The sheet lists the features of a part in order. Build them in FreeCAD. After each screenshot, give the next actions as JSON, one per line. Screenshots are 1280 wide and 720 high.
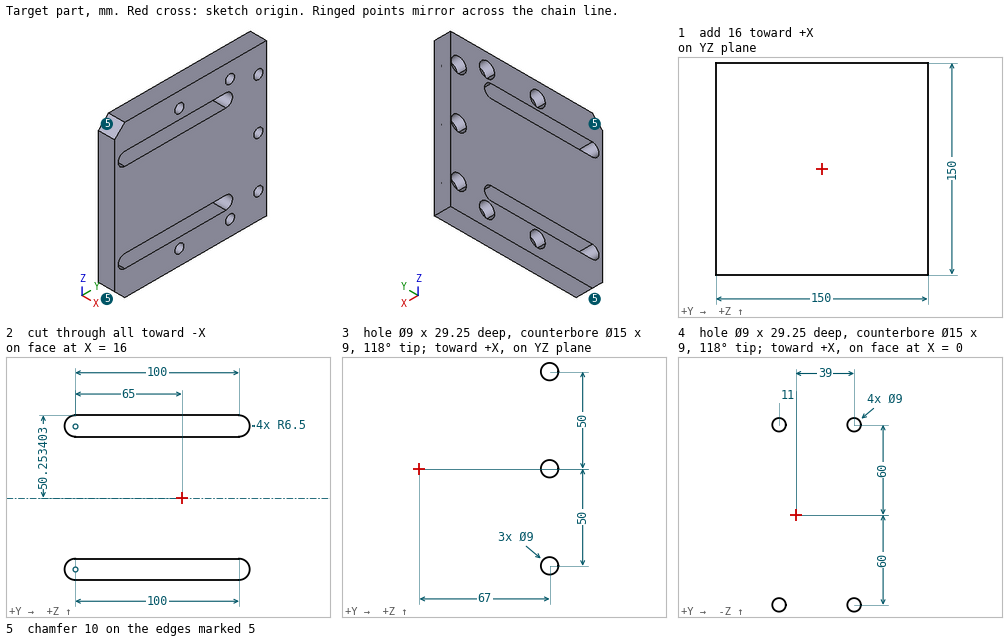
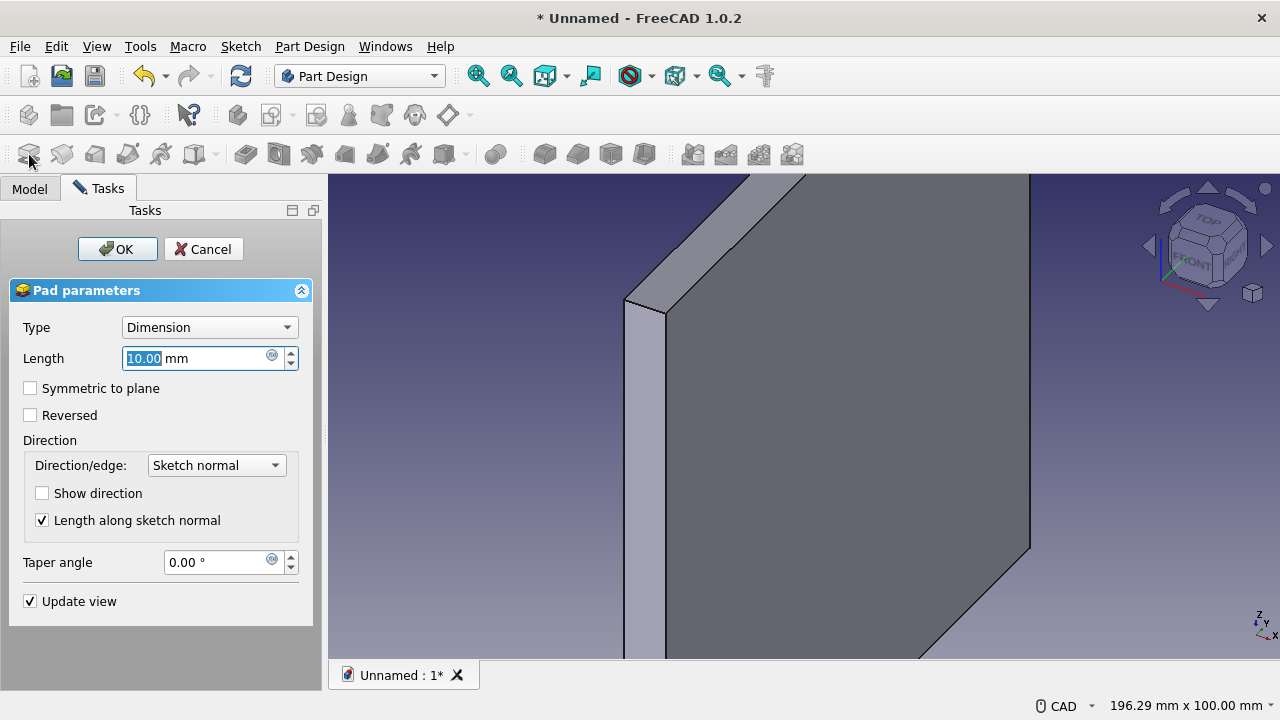
{"action": "type", "text": "16"}
{"action": "key", "text": "Tab"}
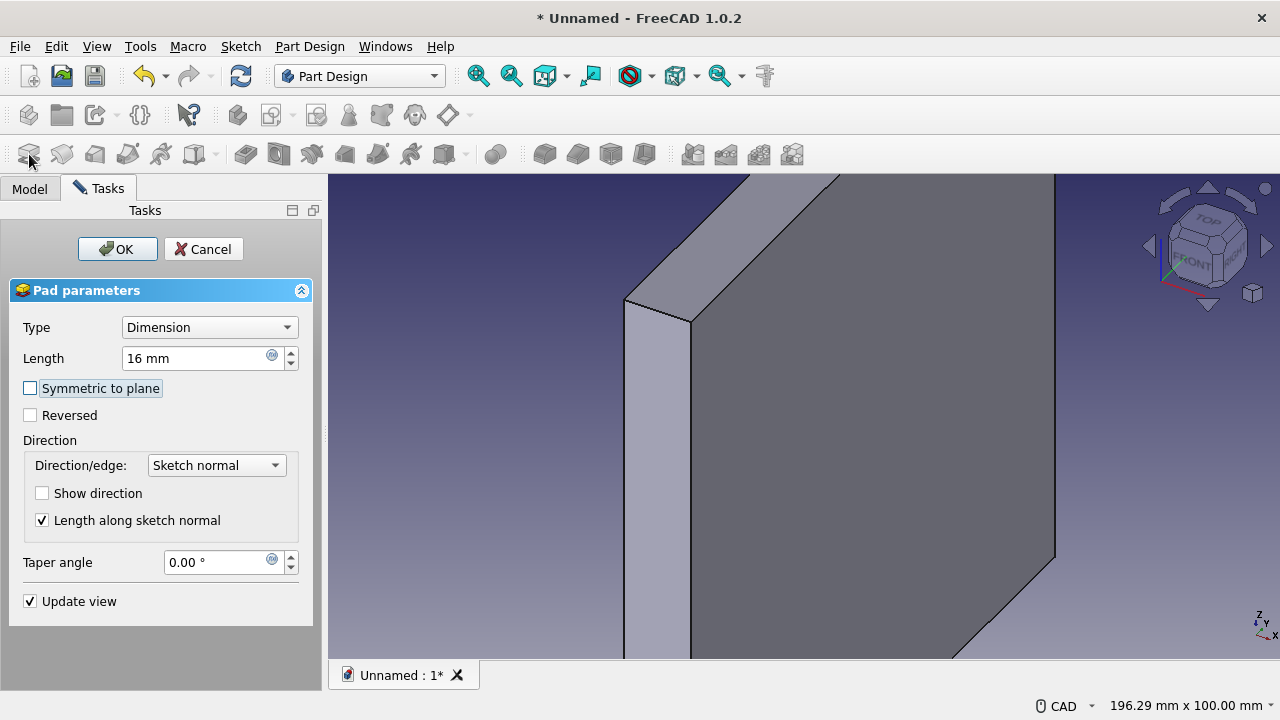
{"action": "left_click", "coordinate": [118, 249]}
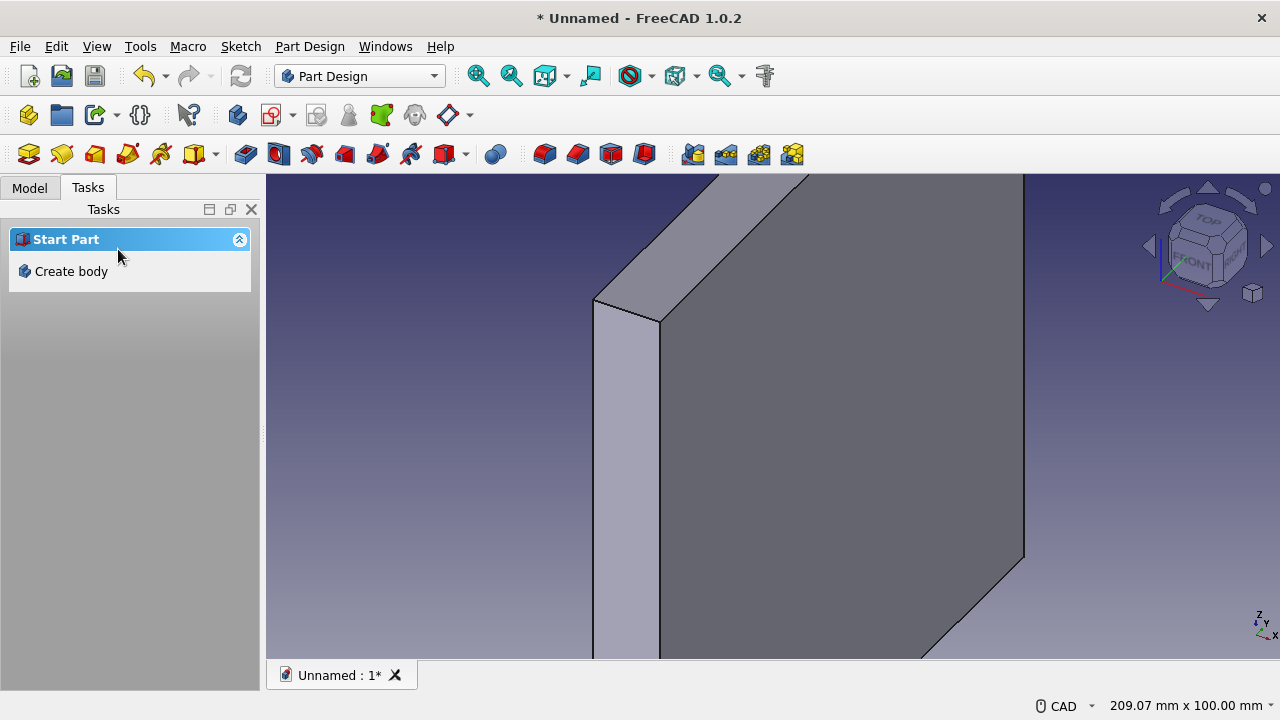
{"action": "left_click", "coordinate": [479, 76]}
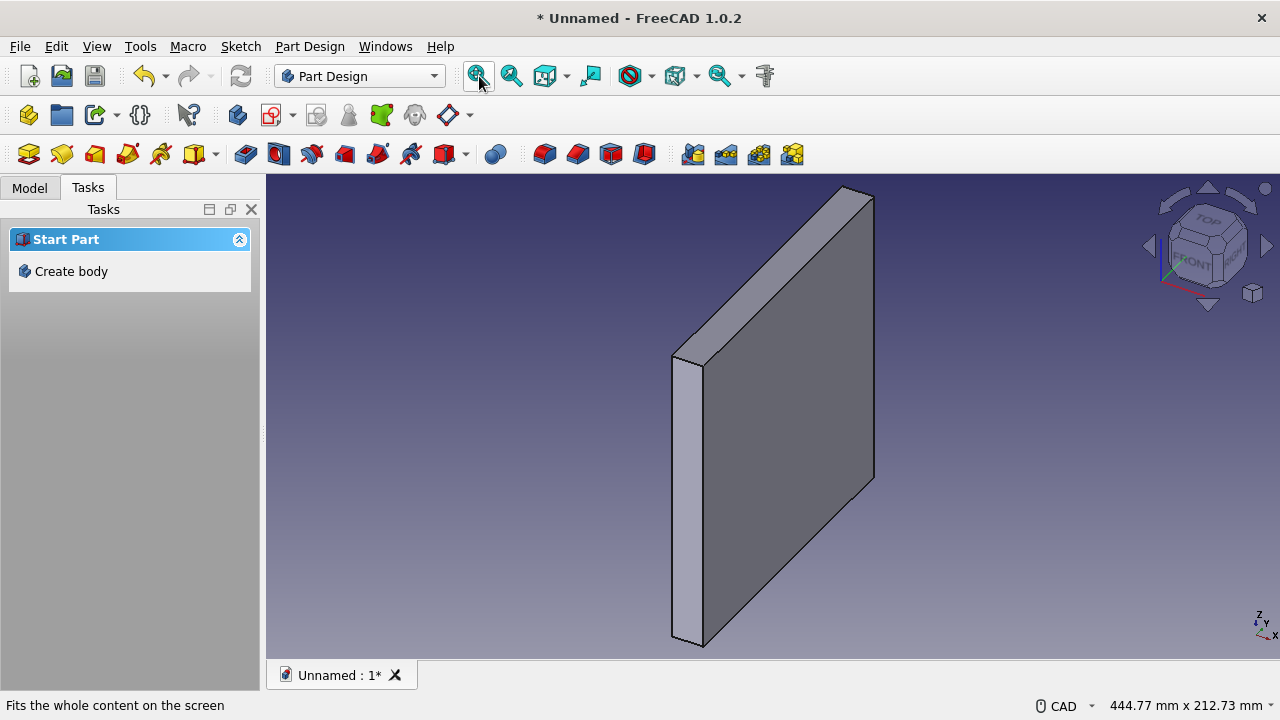
{"action": "left_click", "coordinate": [789, 421]}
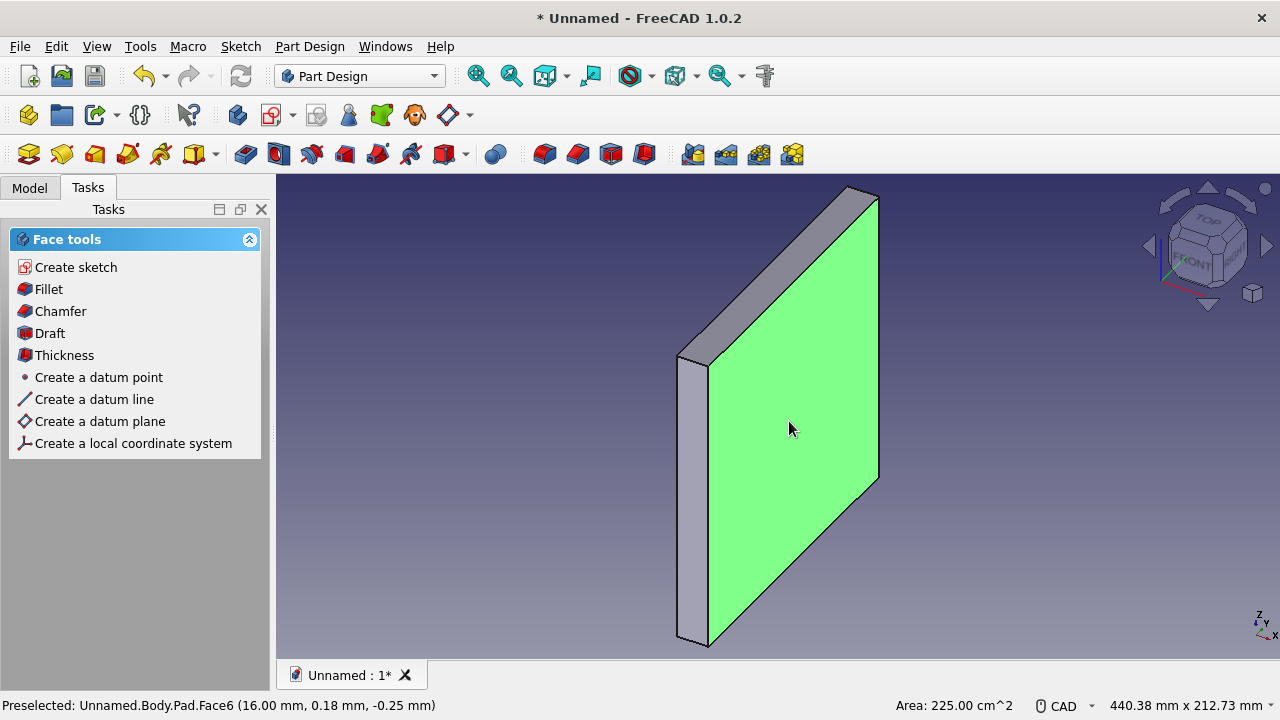
{"action": "left_click", "coordinate": [270, 116]}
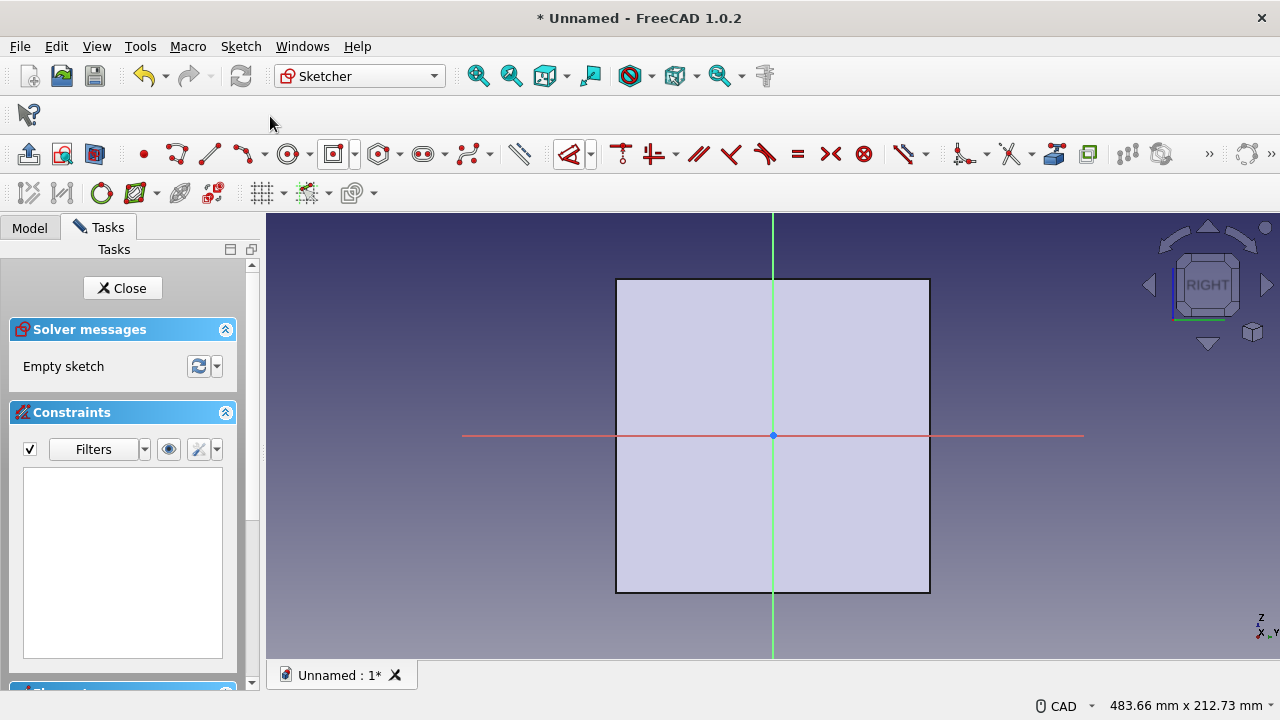
{"action": "left_click", "coordinate": [422, 154]}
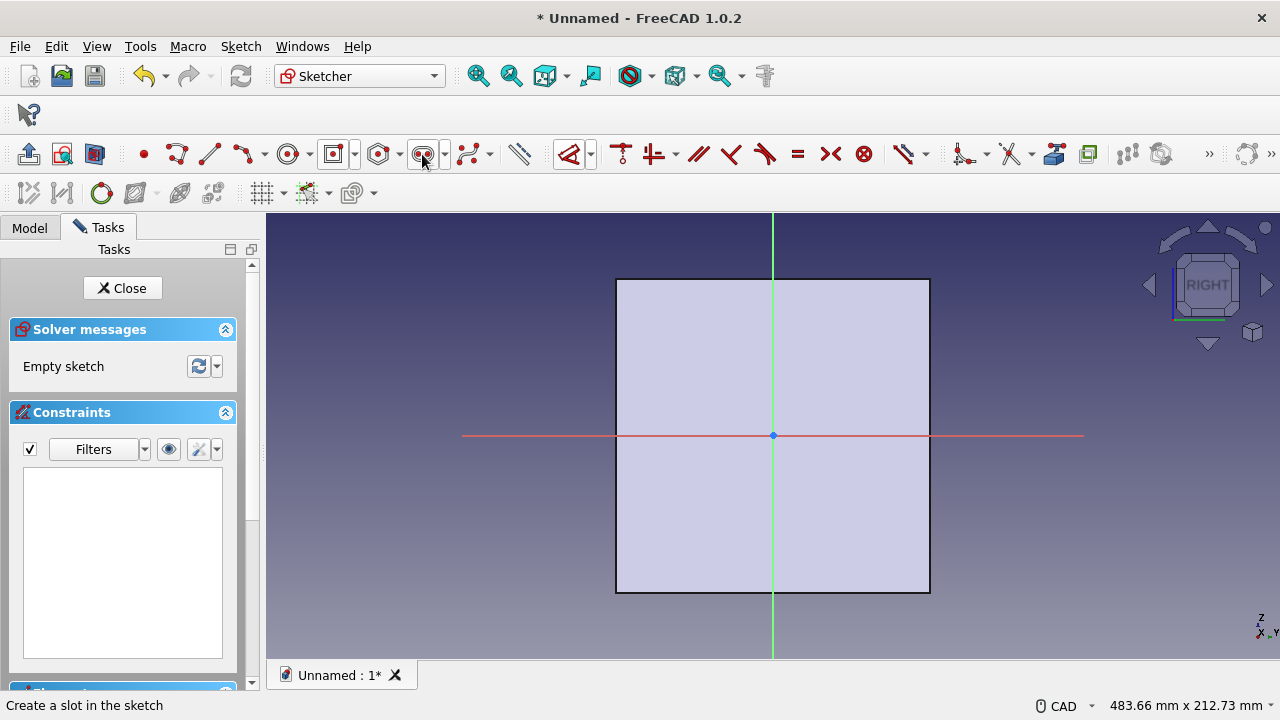
{"action": "scroll", "coordinate": [637, 344], "scroll_direction": "up", "scroll_amount": 3}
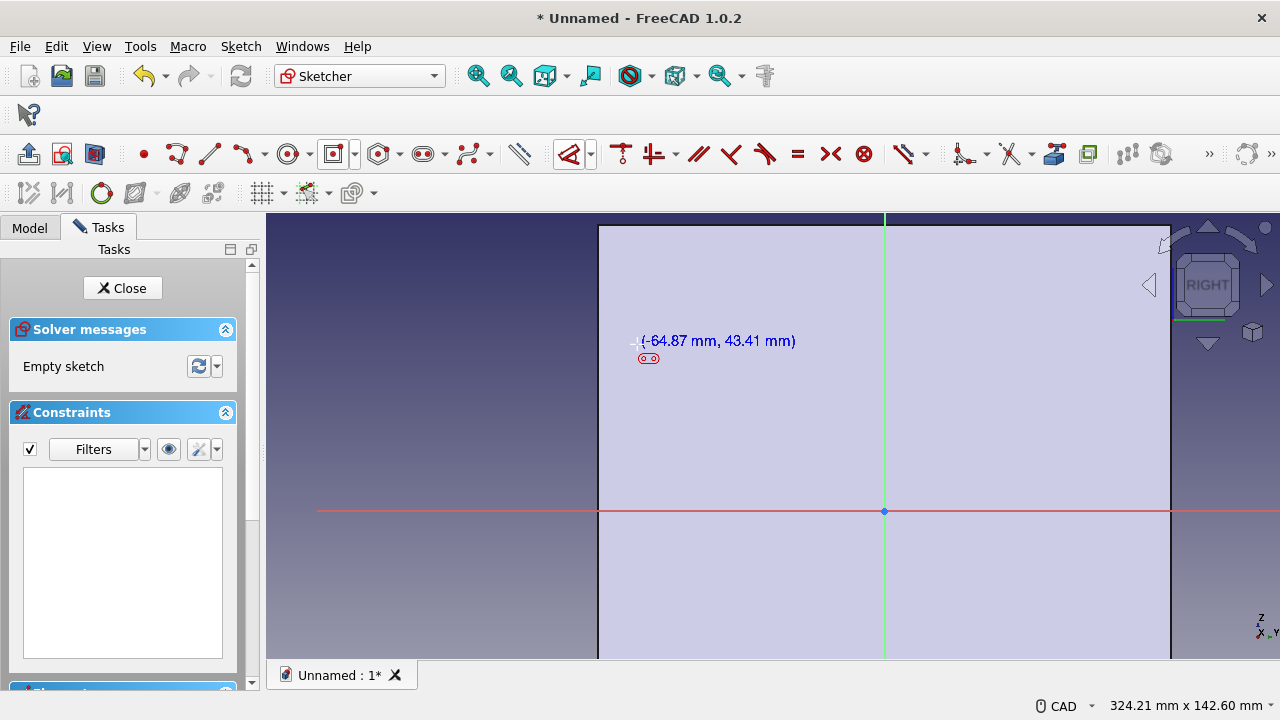
{"action": "left_click", "coordinate": [636, 344]}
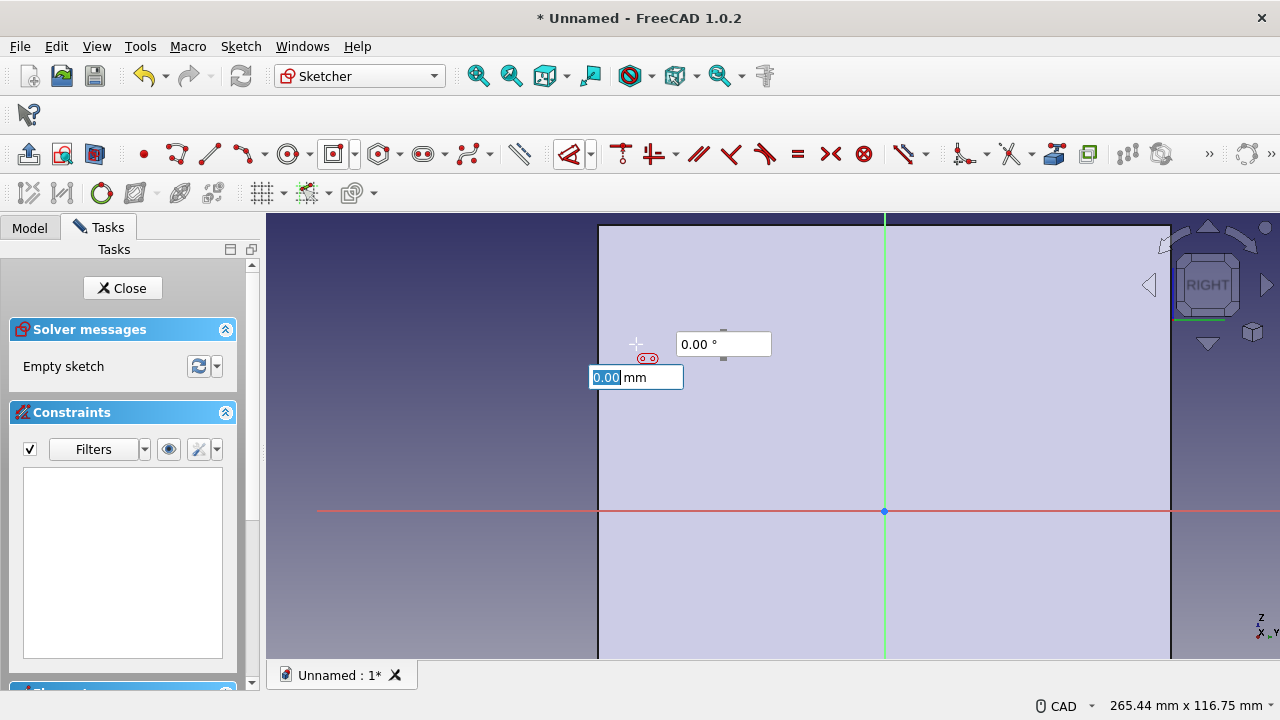
{"action": "left_click", "coordinate": [1018, 344]}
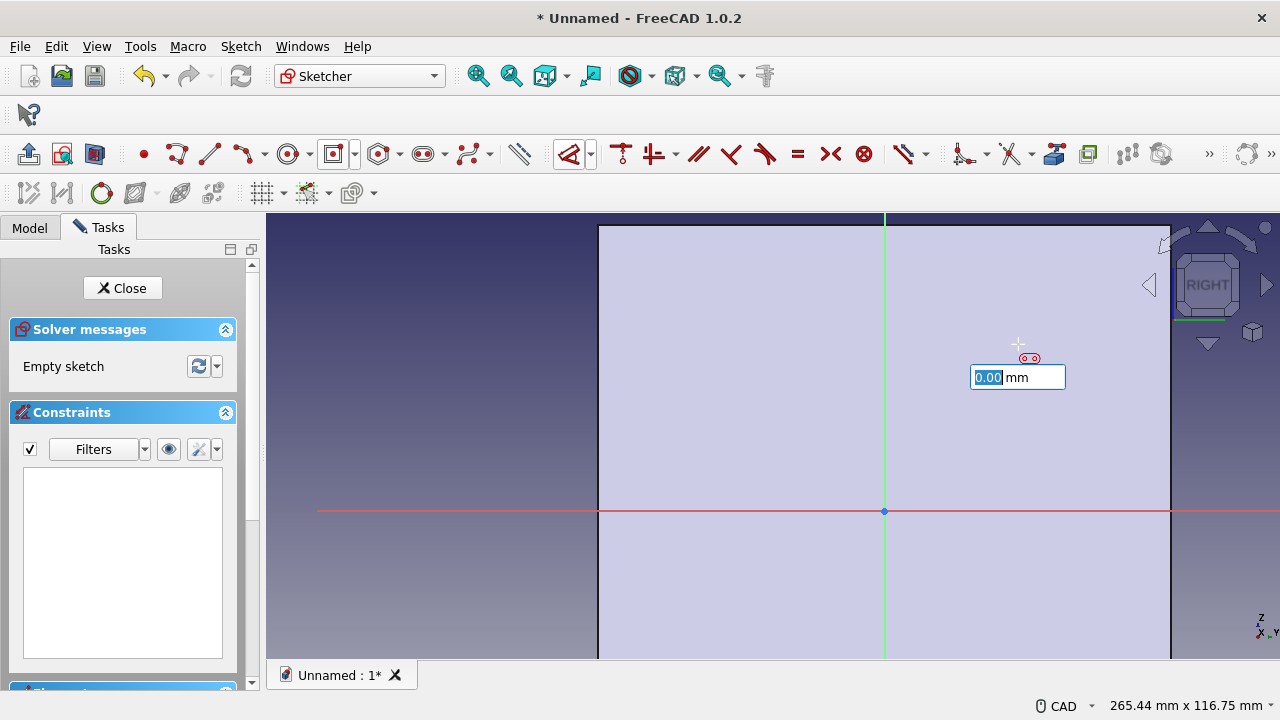
{"action": "left_click", "coordinate": [827, 369]}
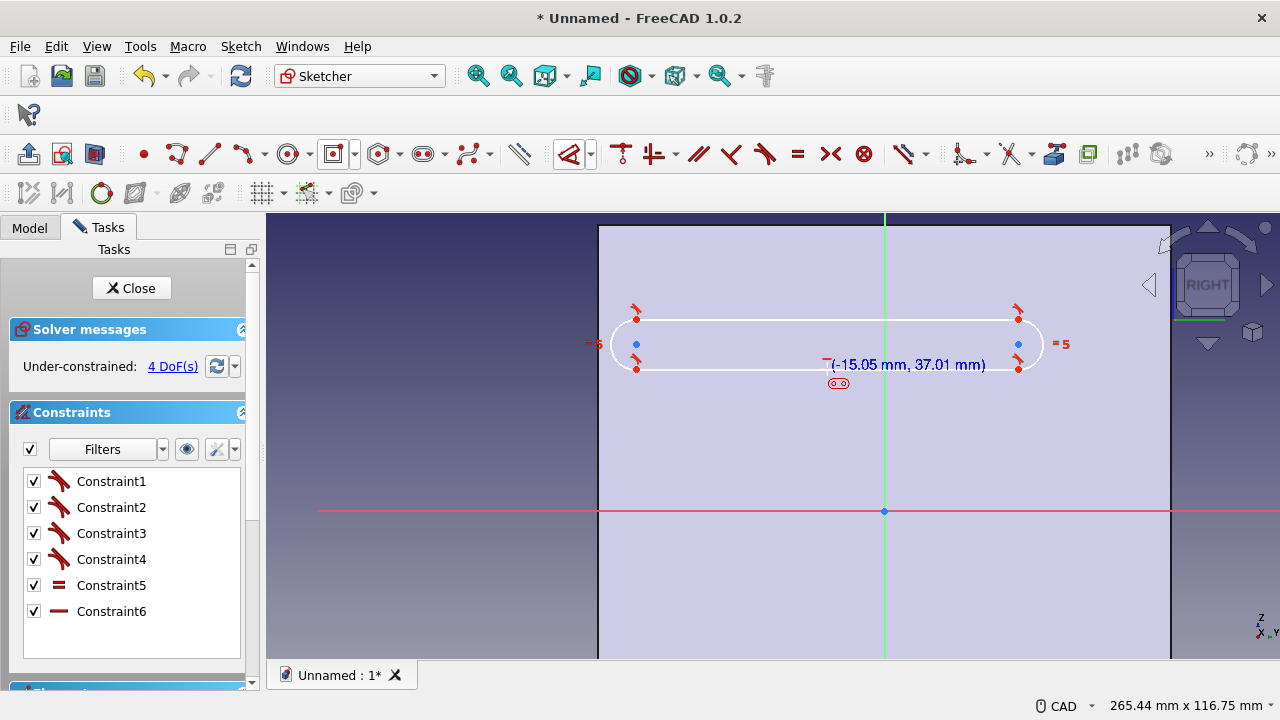
{"action": "scroll", "coordinate": [455, 283], "scroll_direction": "down", "scroll_amount": 2}